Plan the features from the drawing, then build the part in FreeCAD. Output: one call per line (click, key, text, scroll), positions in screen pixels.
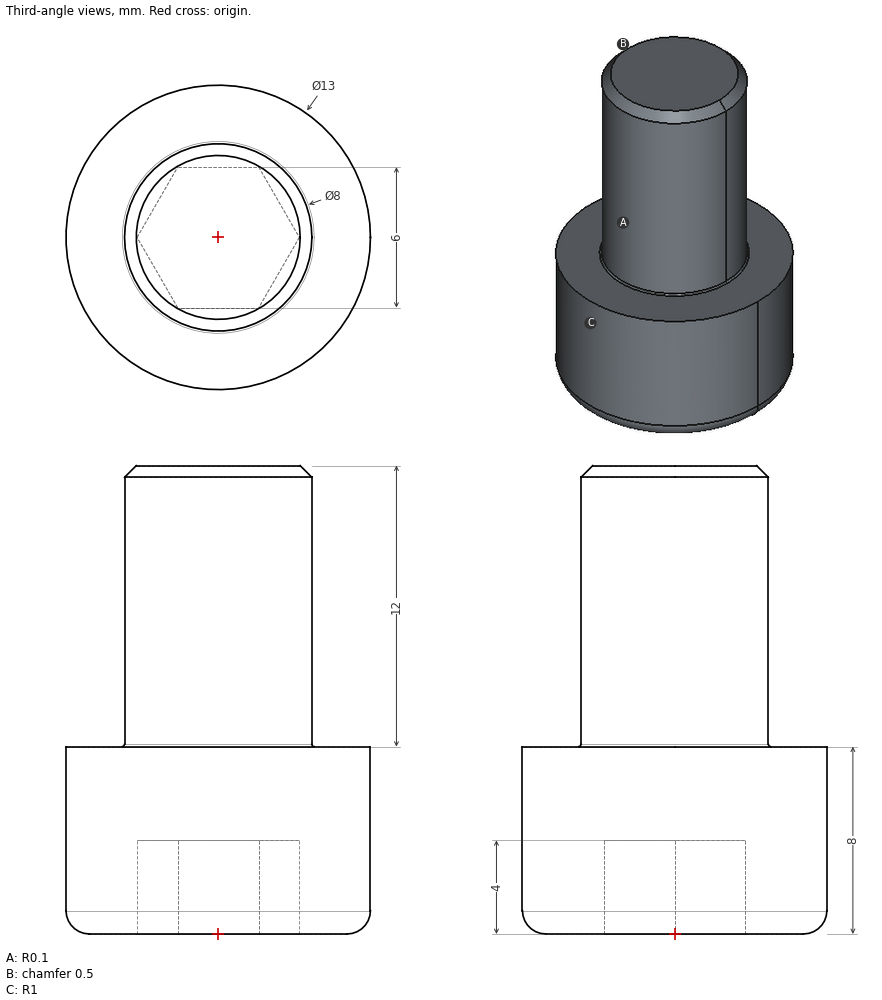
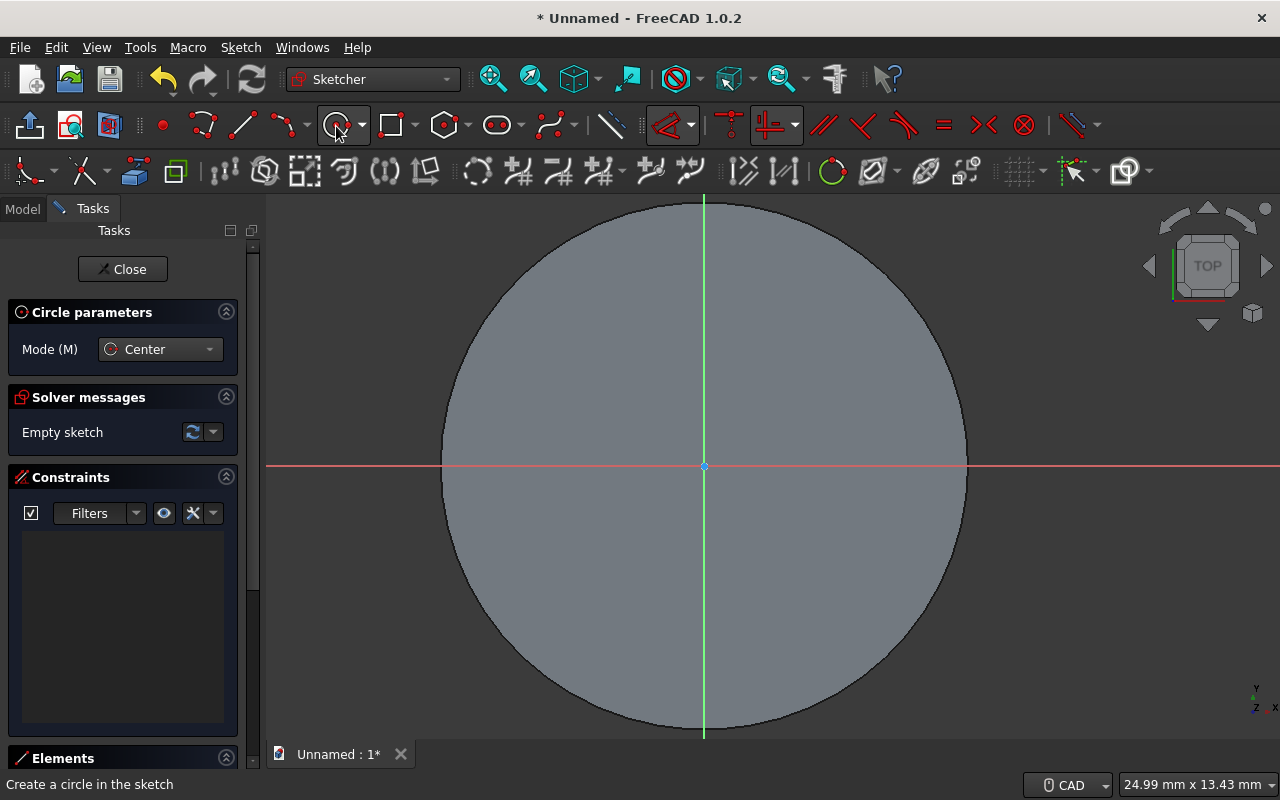
click(704, 466)
click(819, 351)
key(Escape)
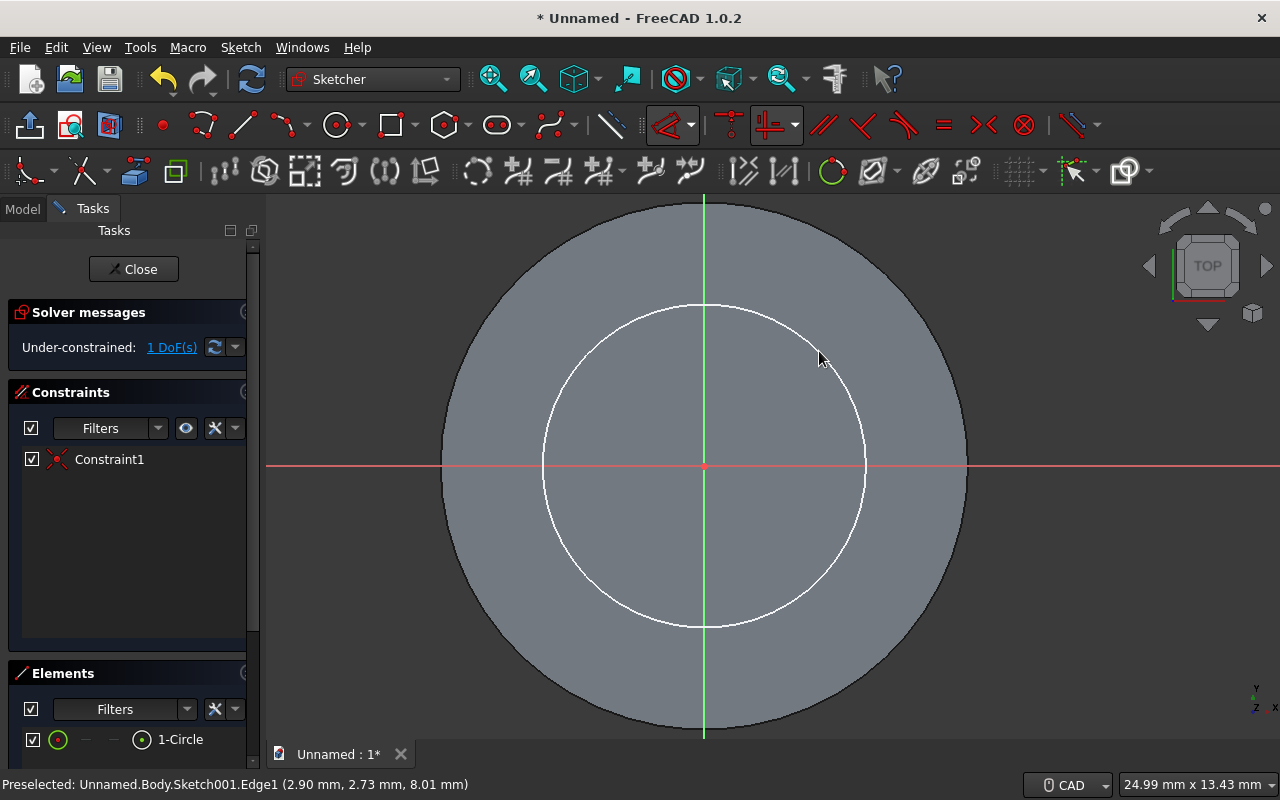
click(818, 351)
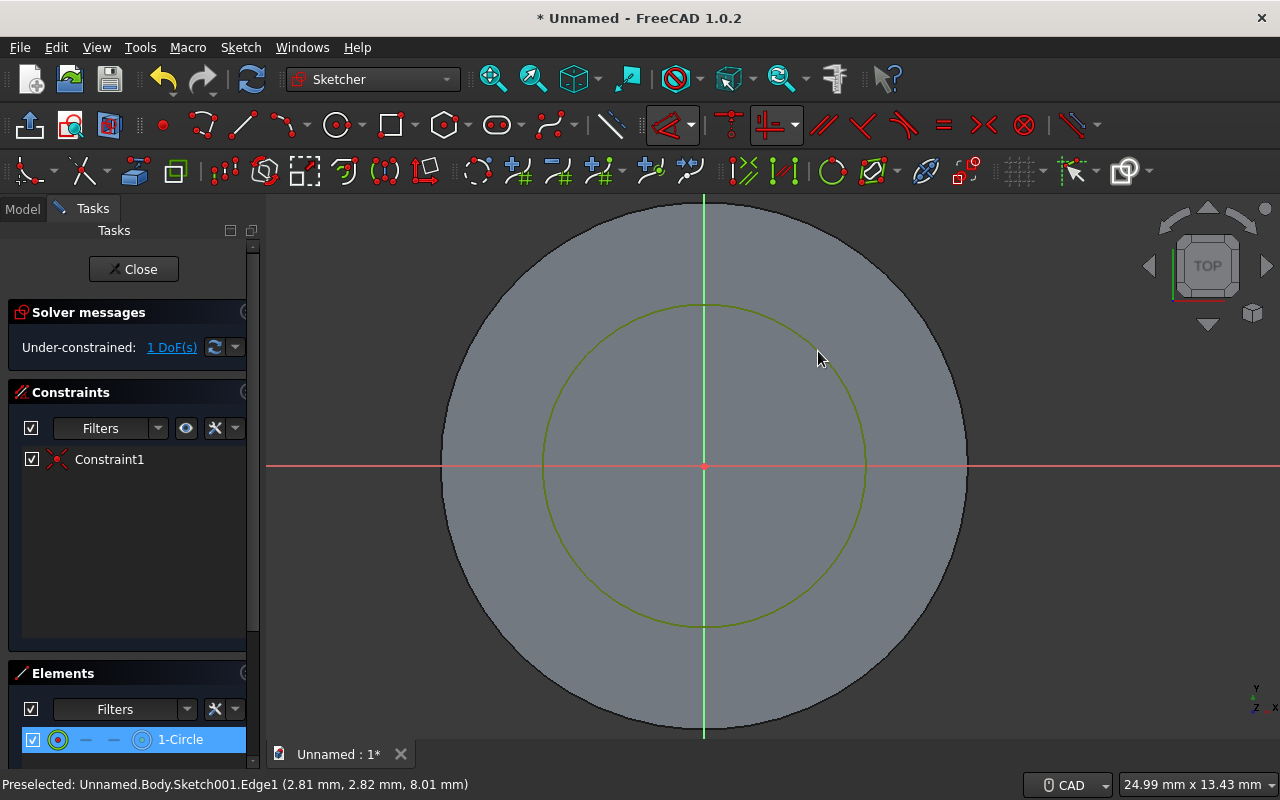
click(694, 126)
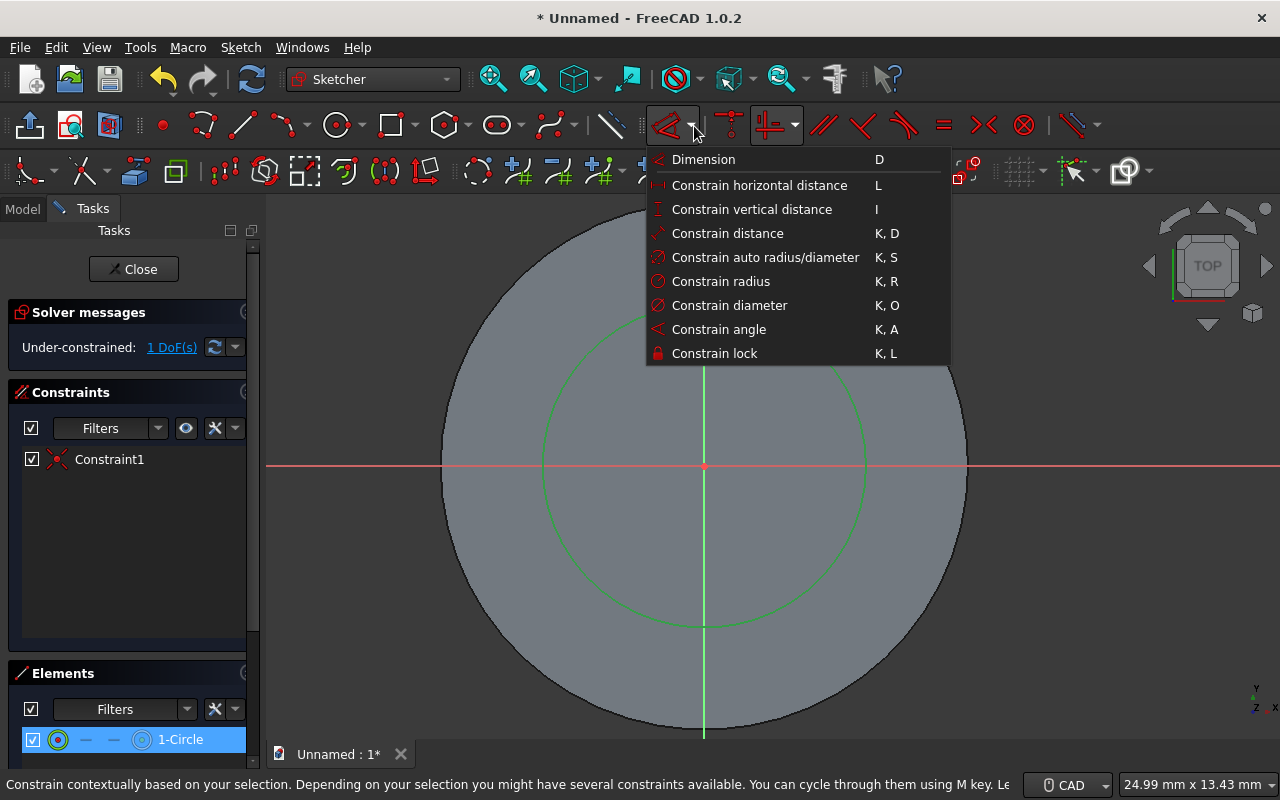
click(799, 305)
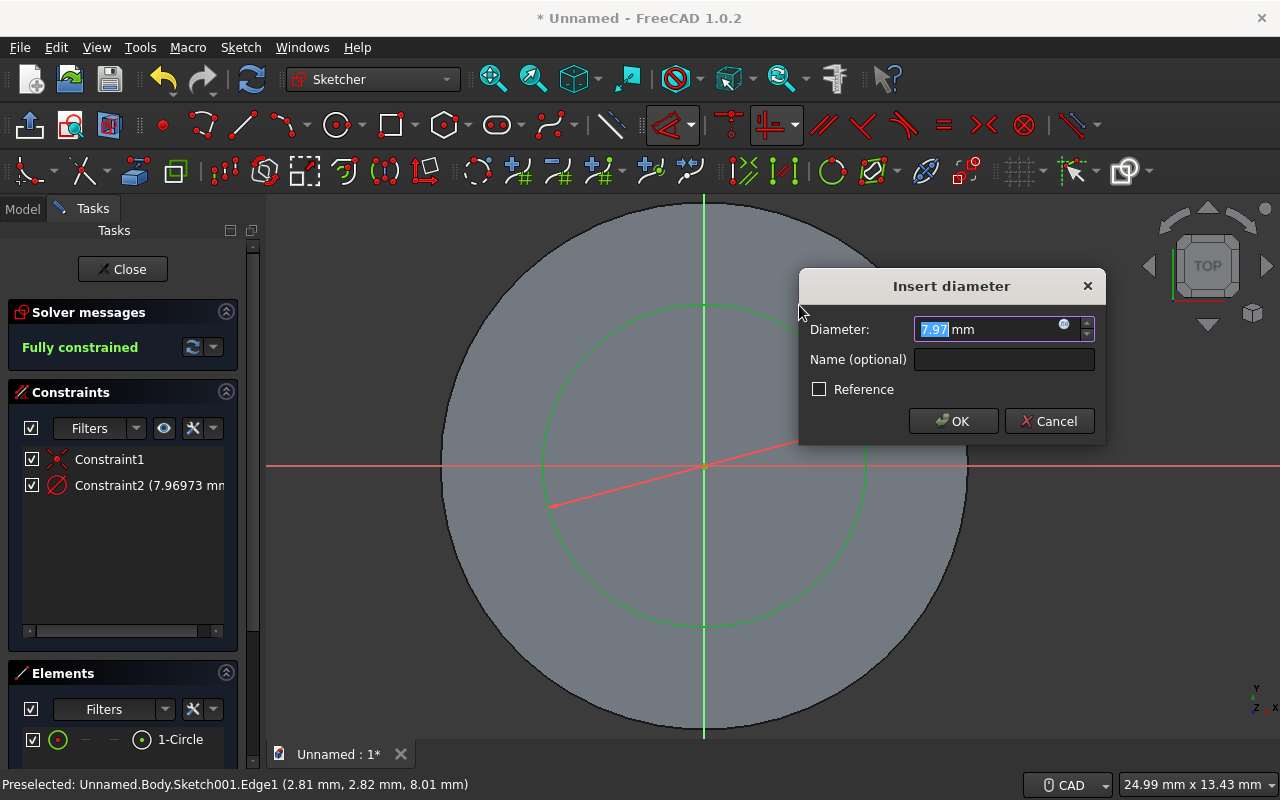
text(8)
key(Return)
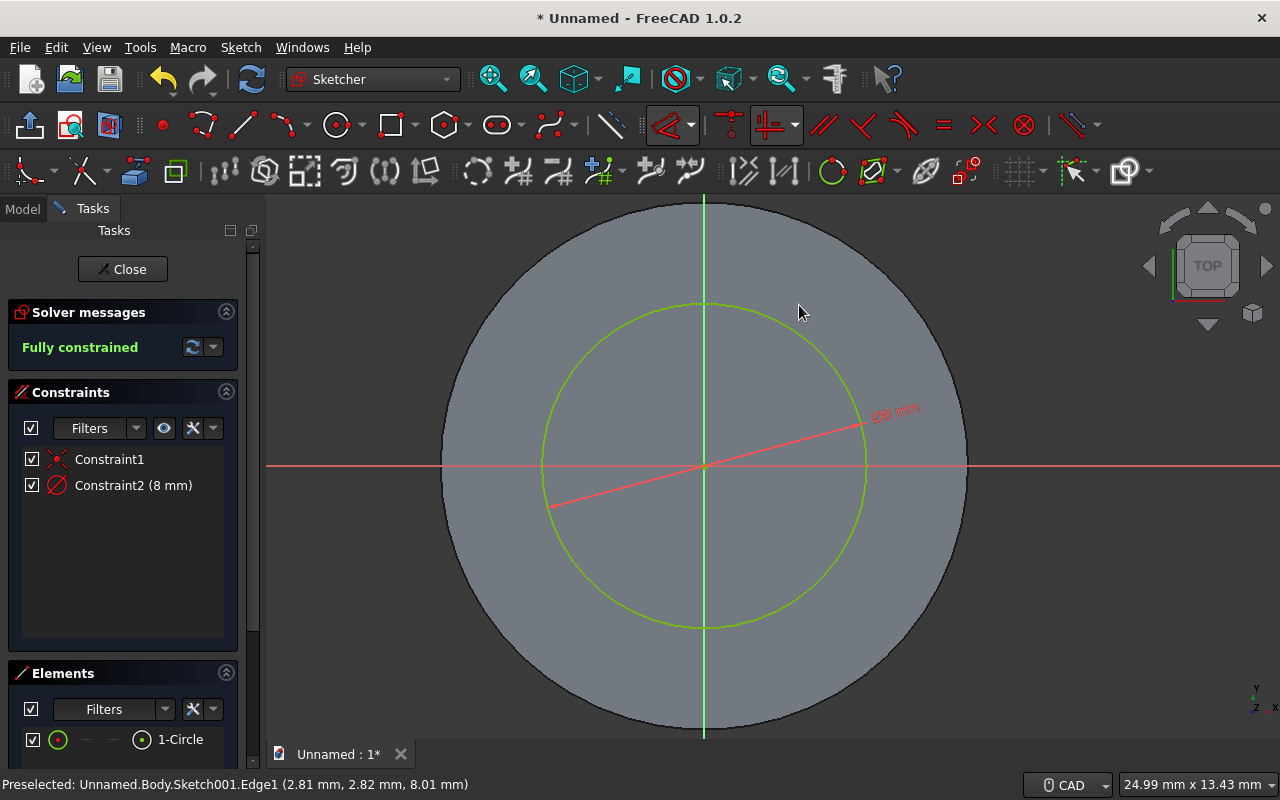
click(123, 269)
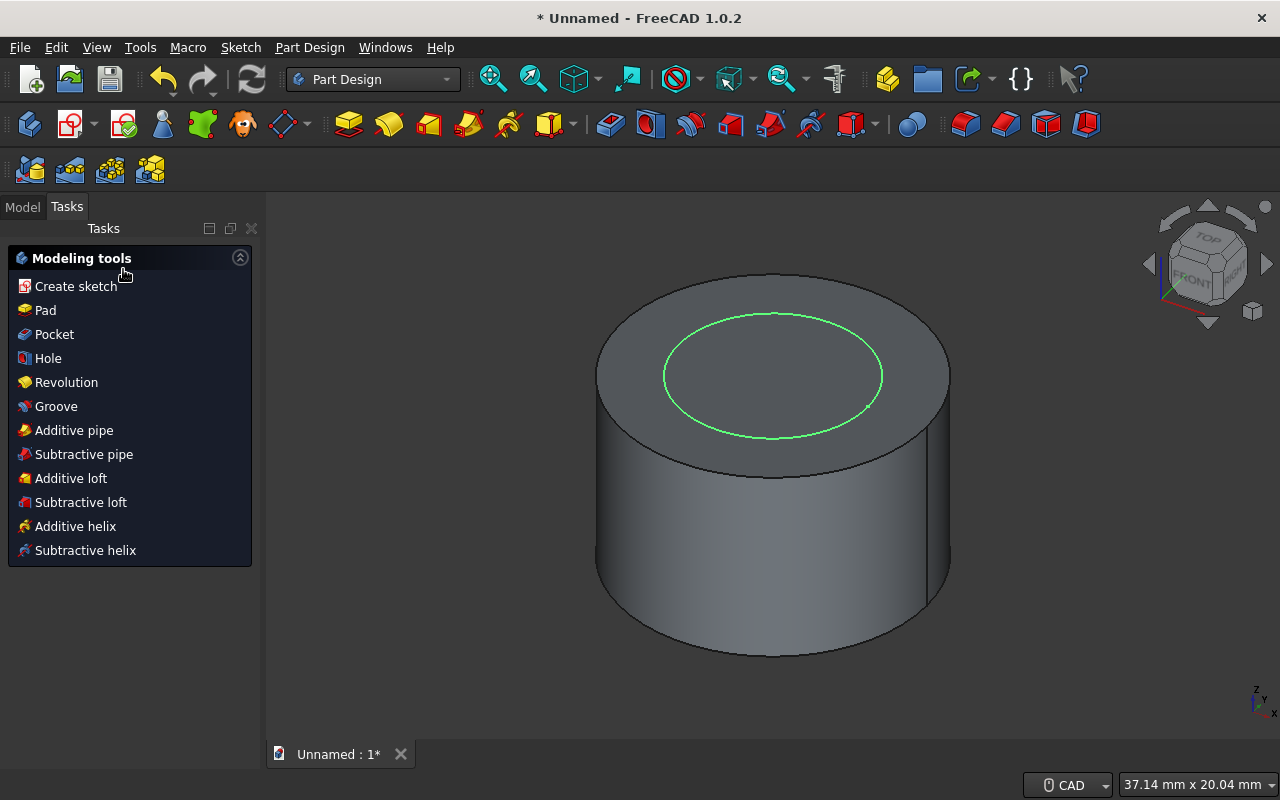
click(350, 124)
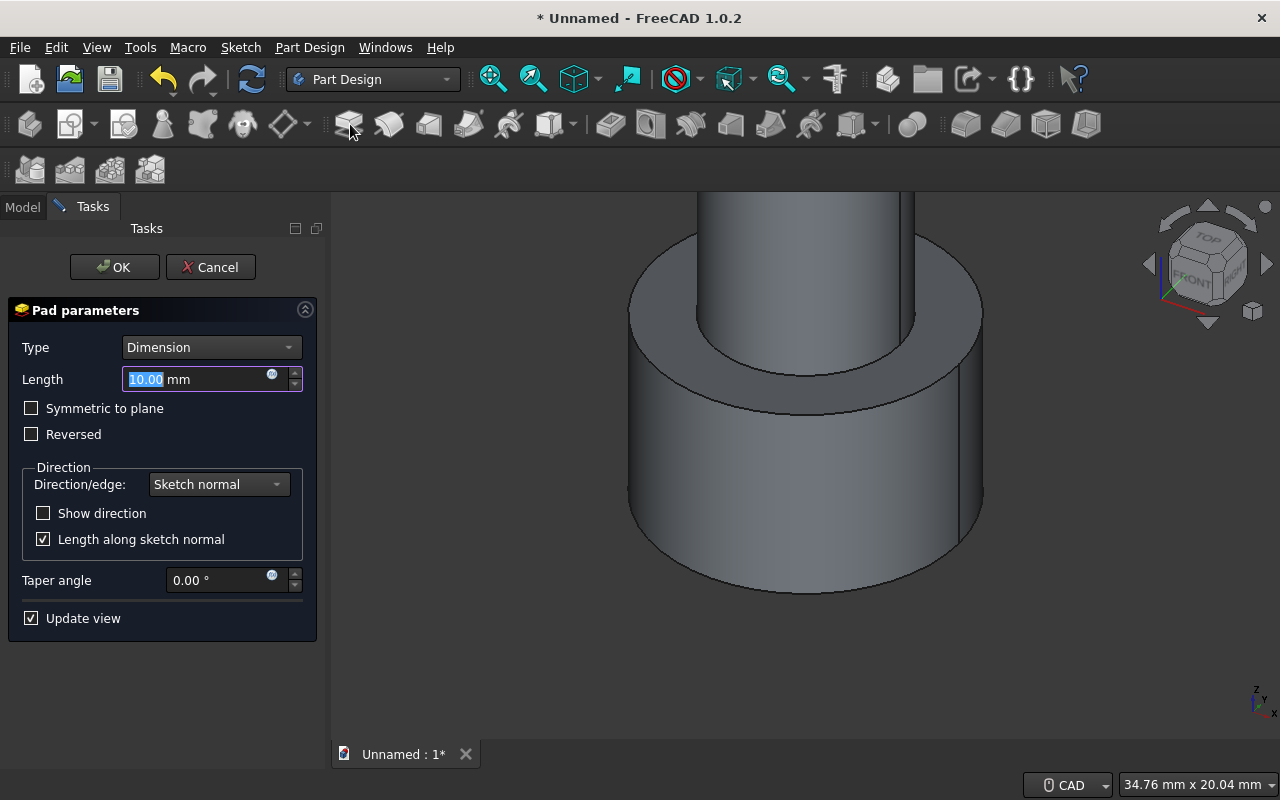
text(12)
key(Tab)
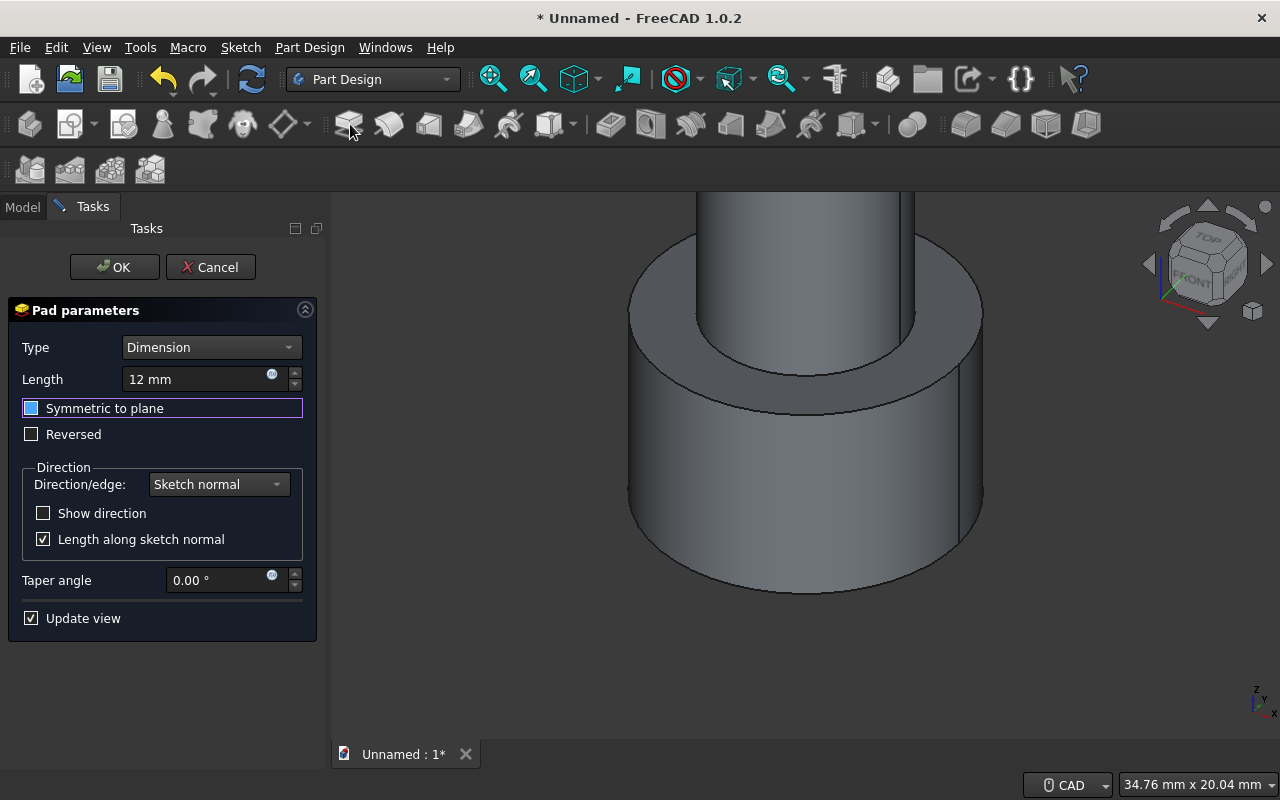
click(115, 267)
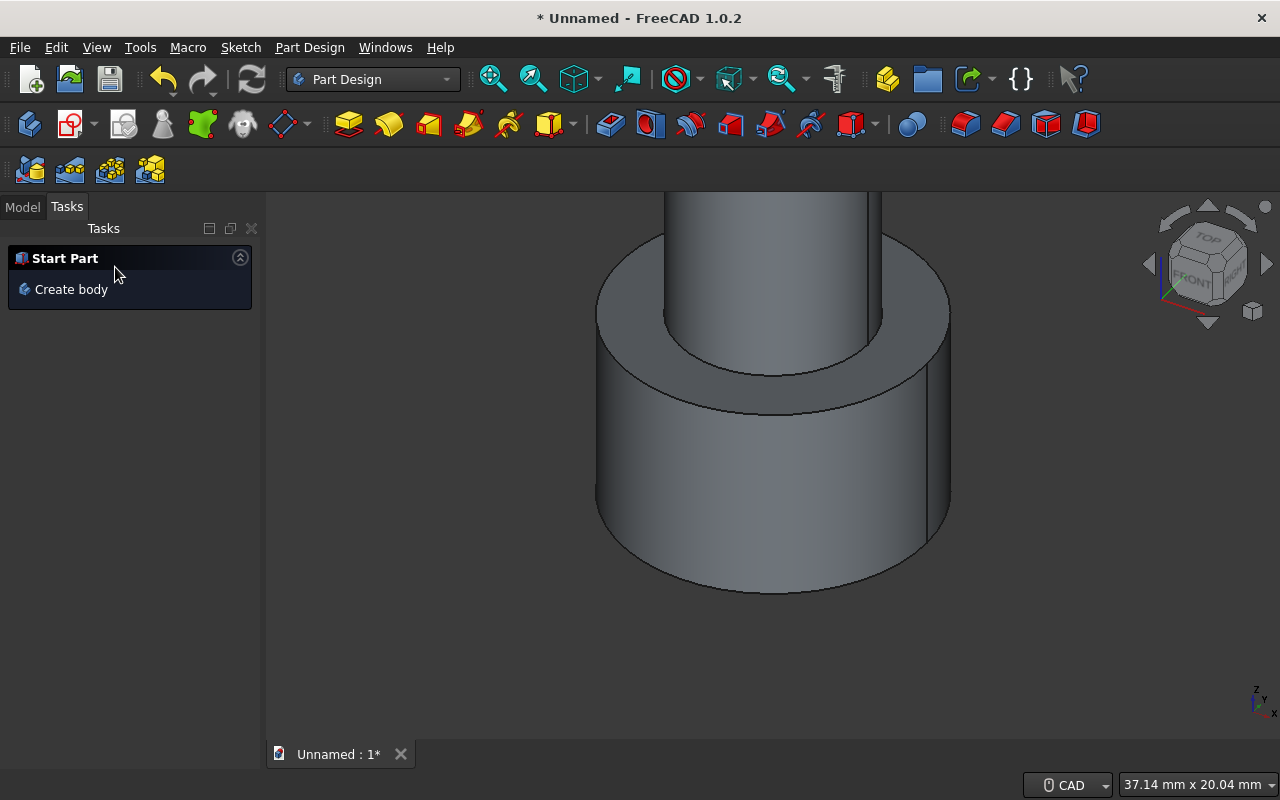
click(494, 80)